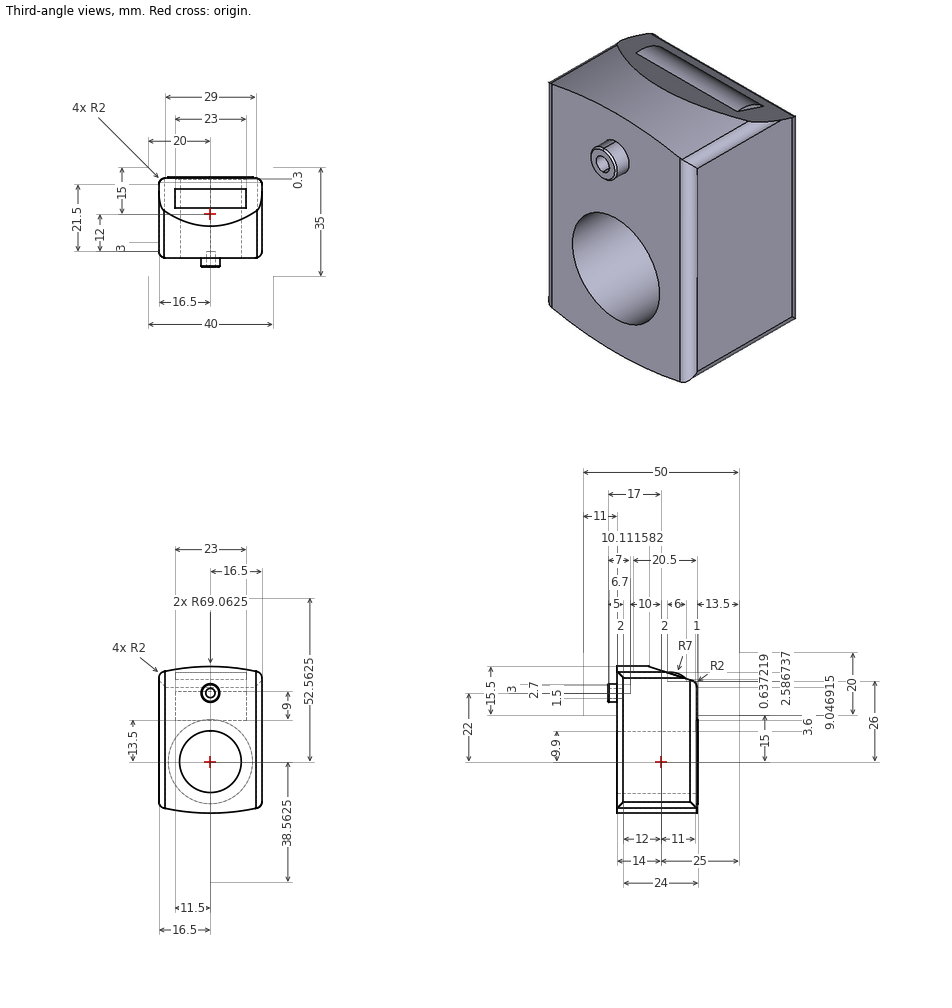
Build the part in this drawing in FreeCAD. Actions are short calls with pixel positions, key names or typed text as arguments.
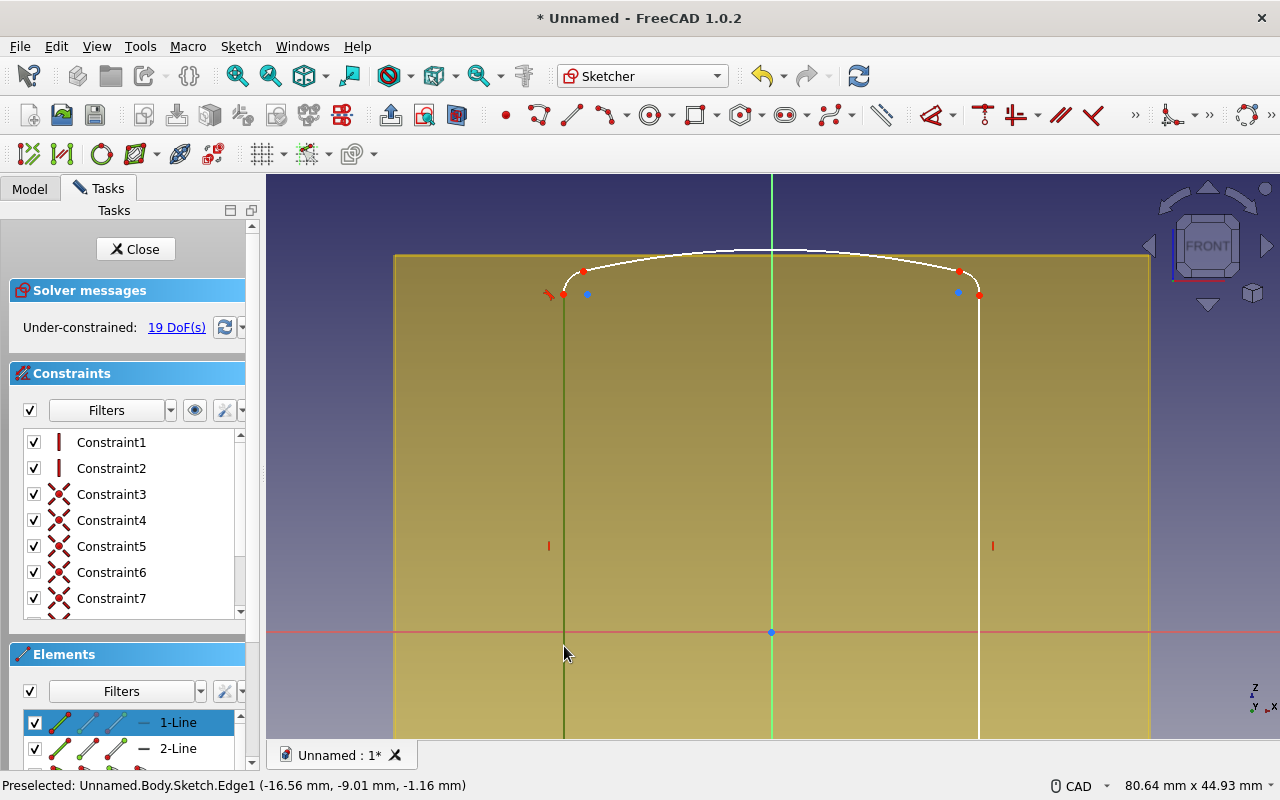
scroll(567, 278, down, 2)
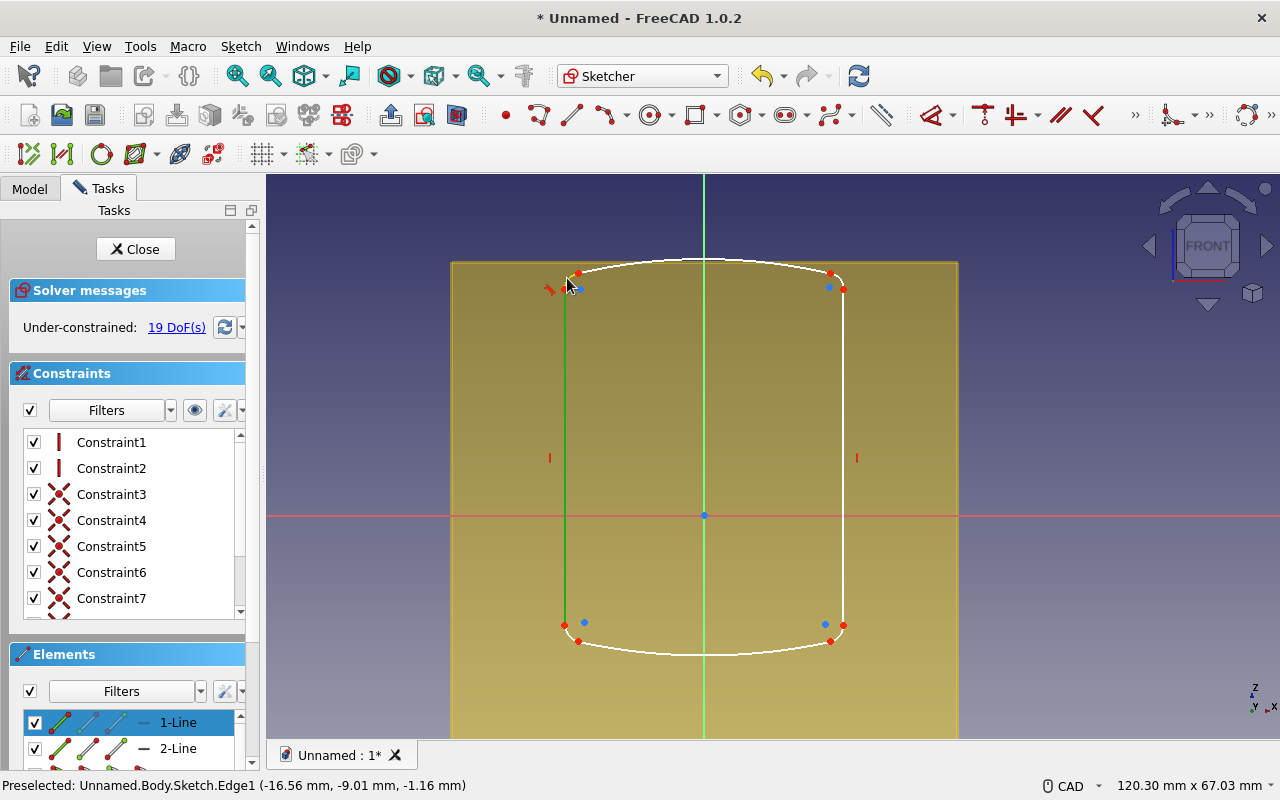
scroll(567, 632, up, 4)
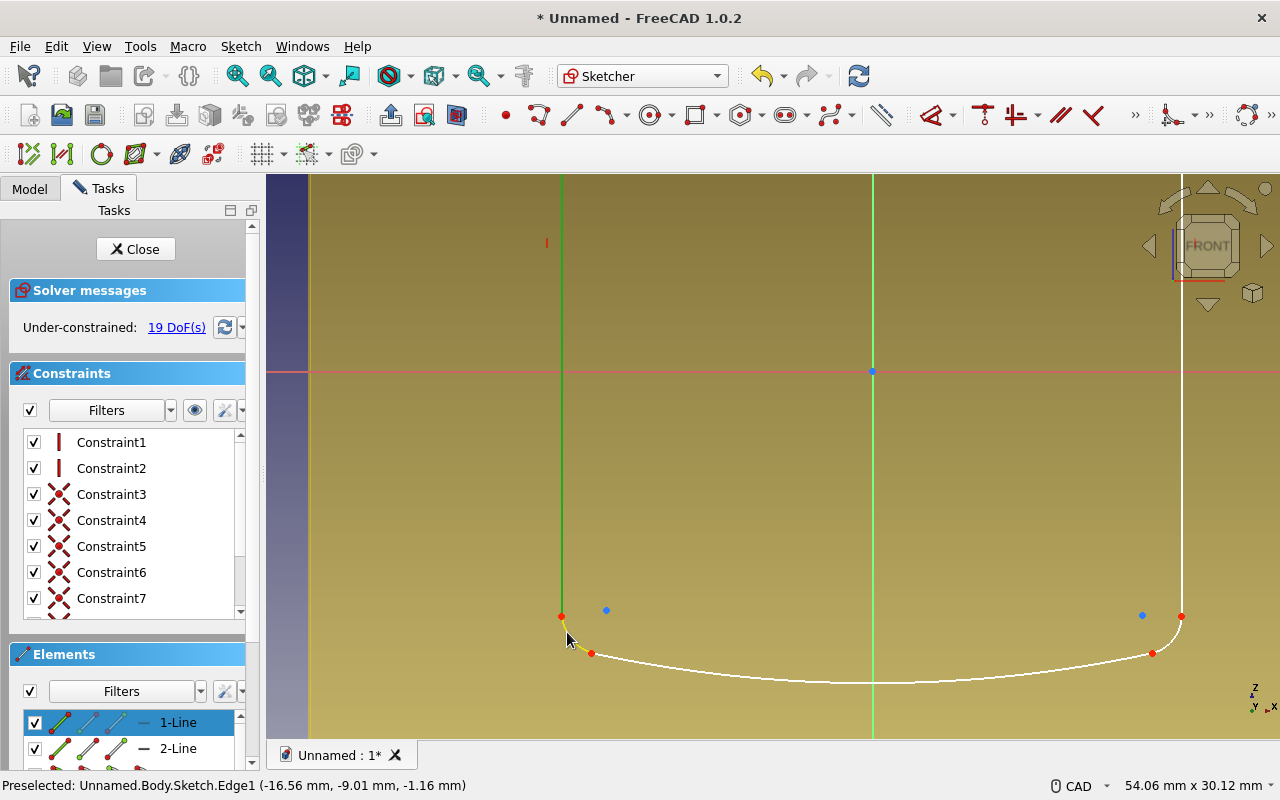
click(566, 631)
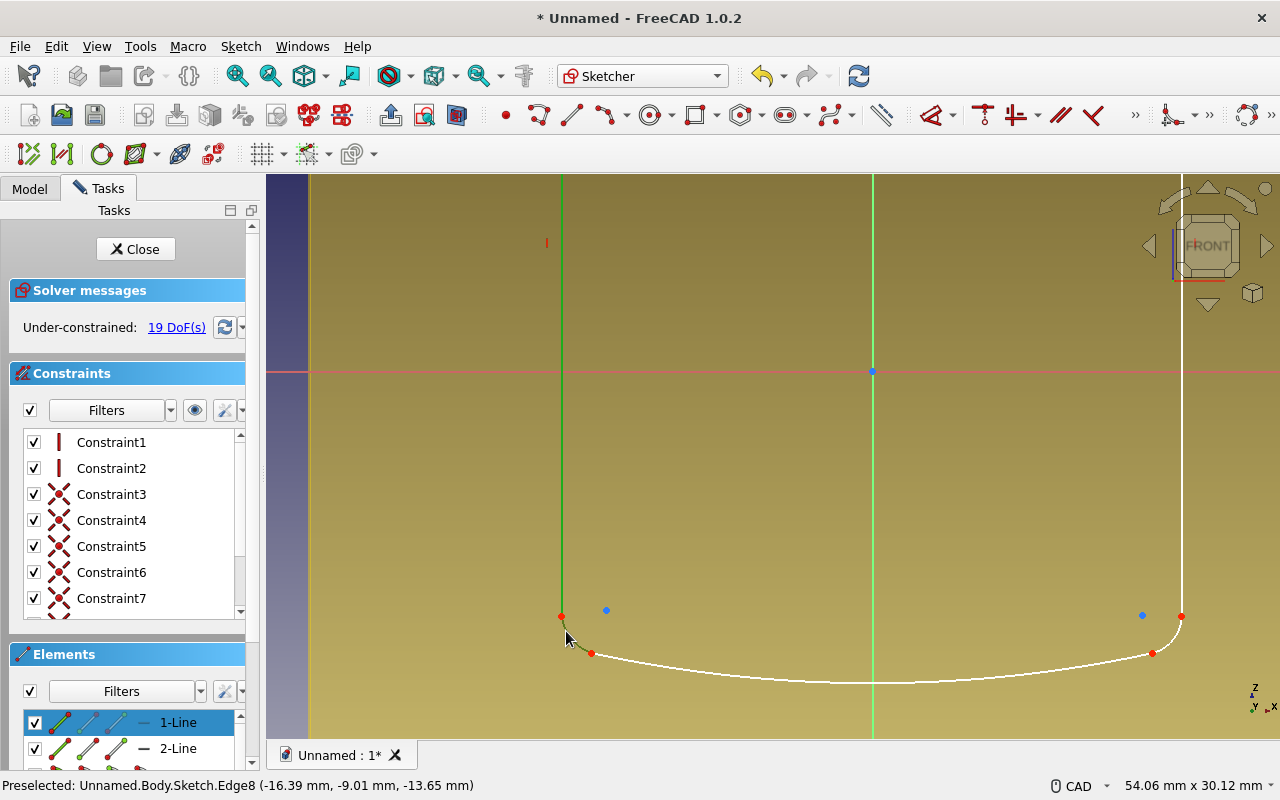
key(t)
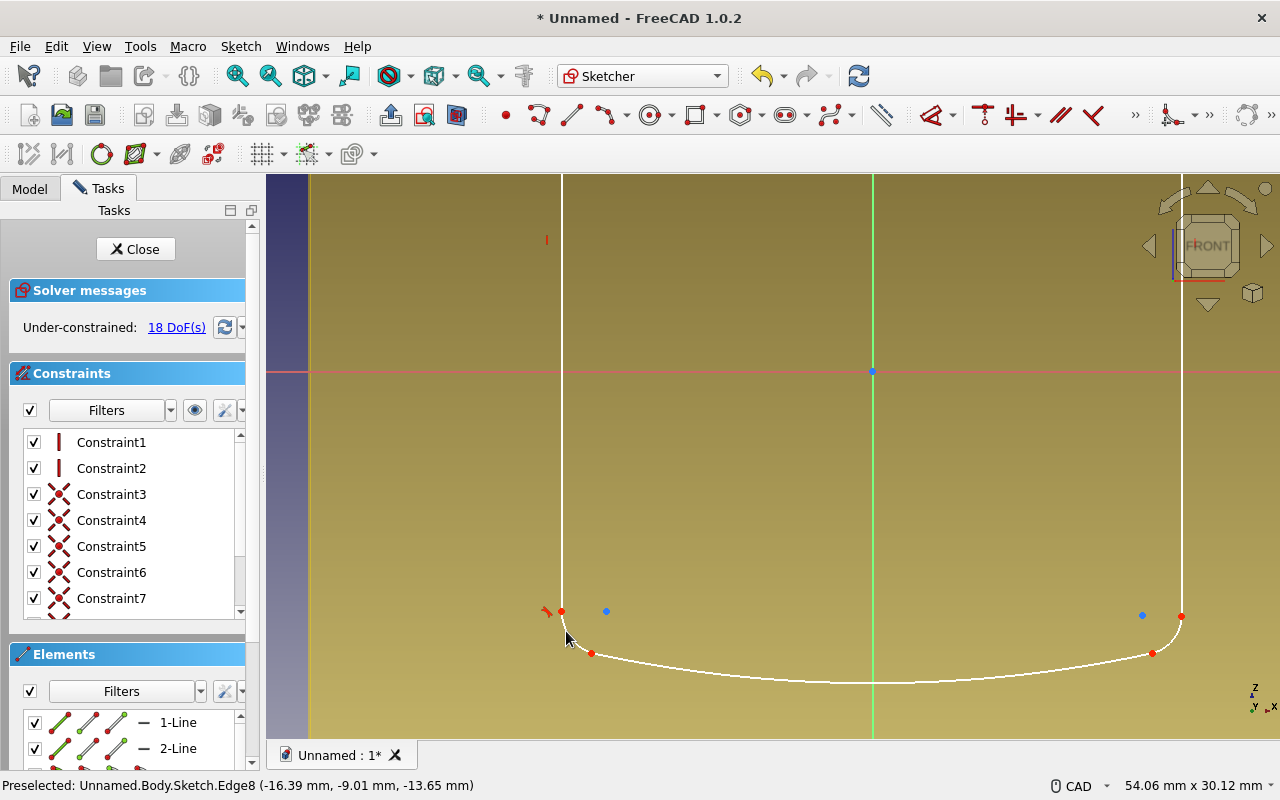
scroll(567, 633, down, 4)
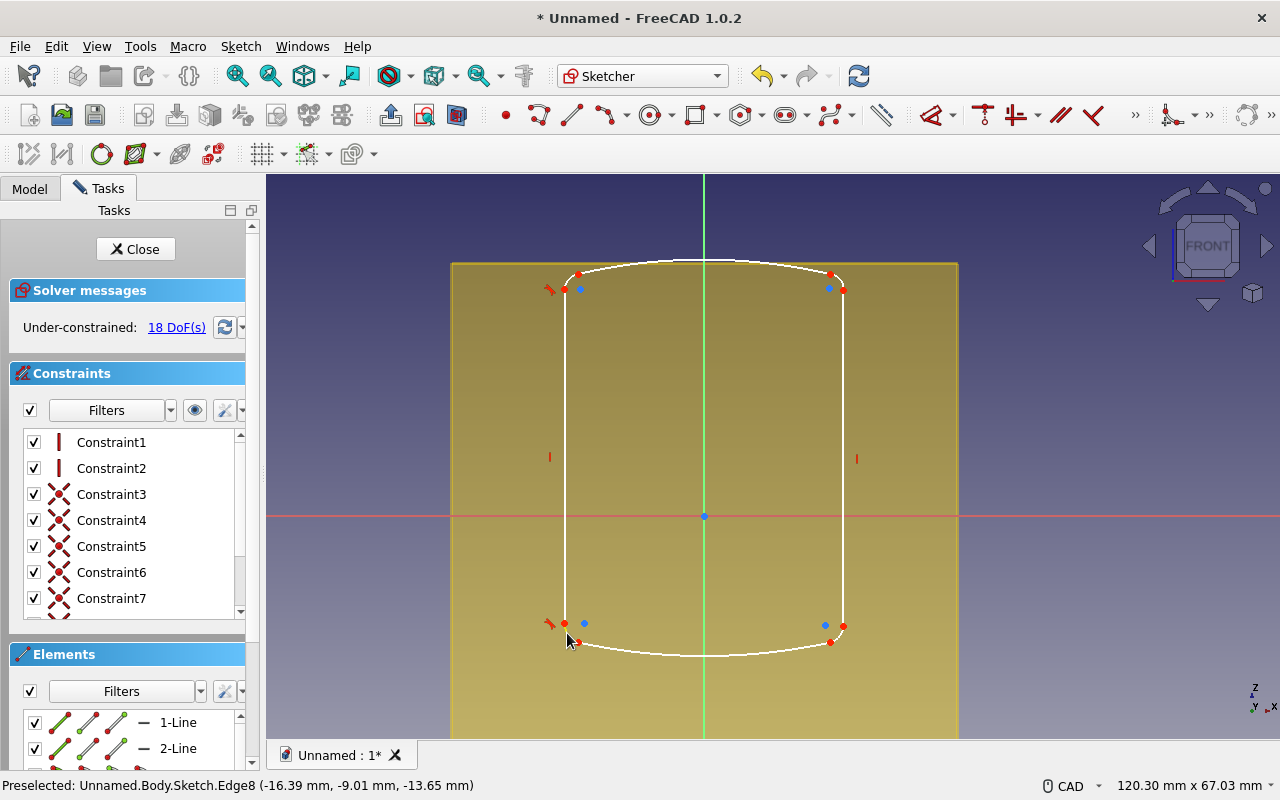
click(843, 391)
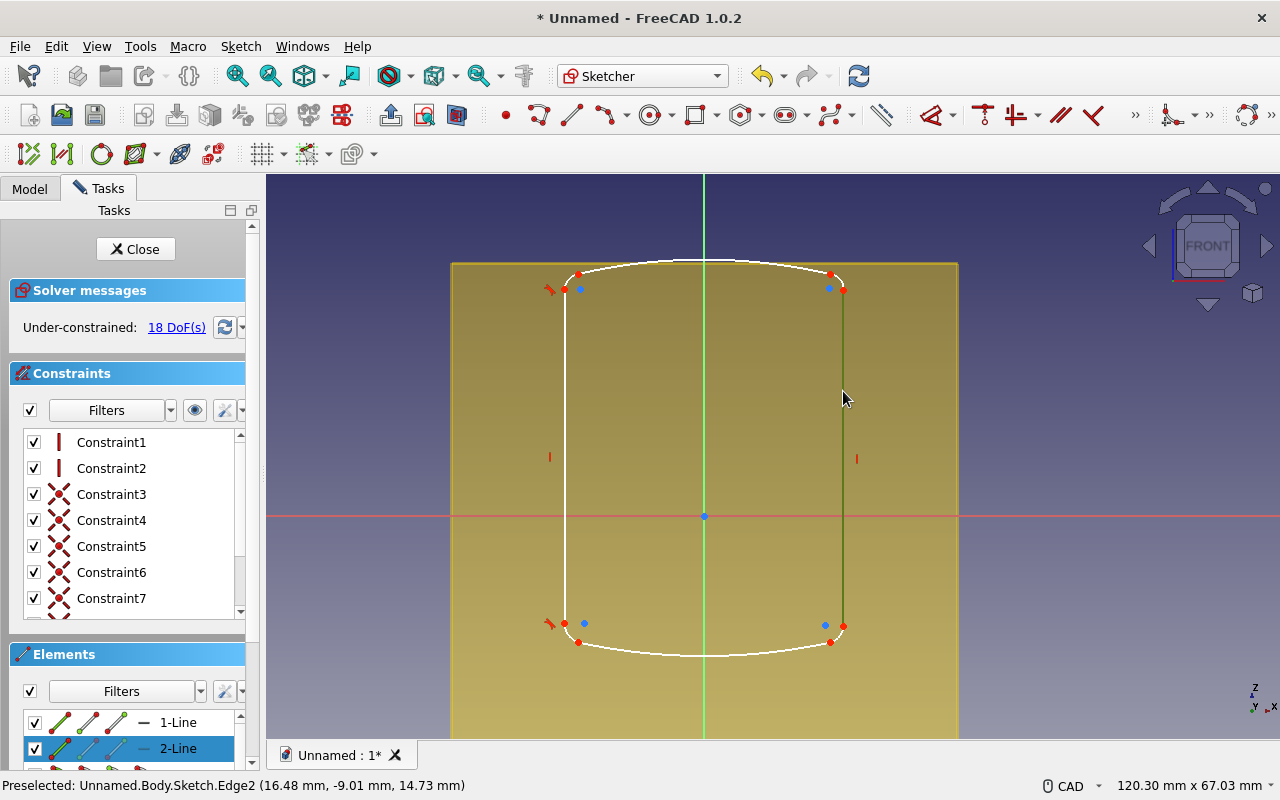
scroll(840, 279, up, 2)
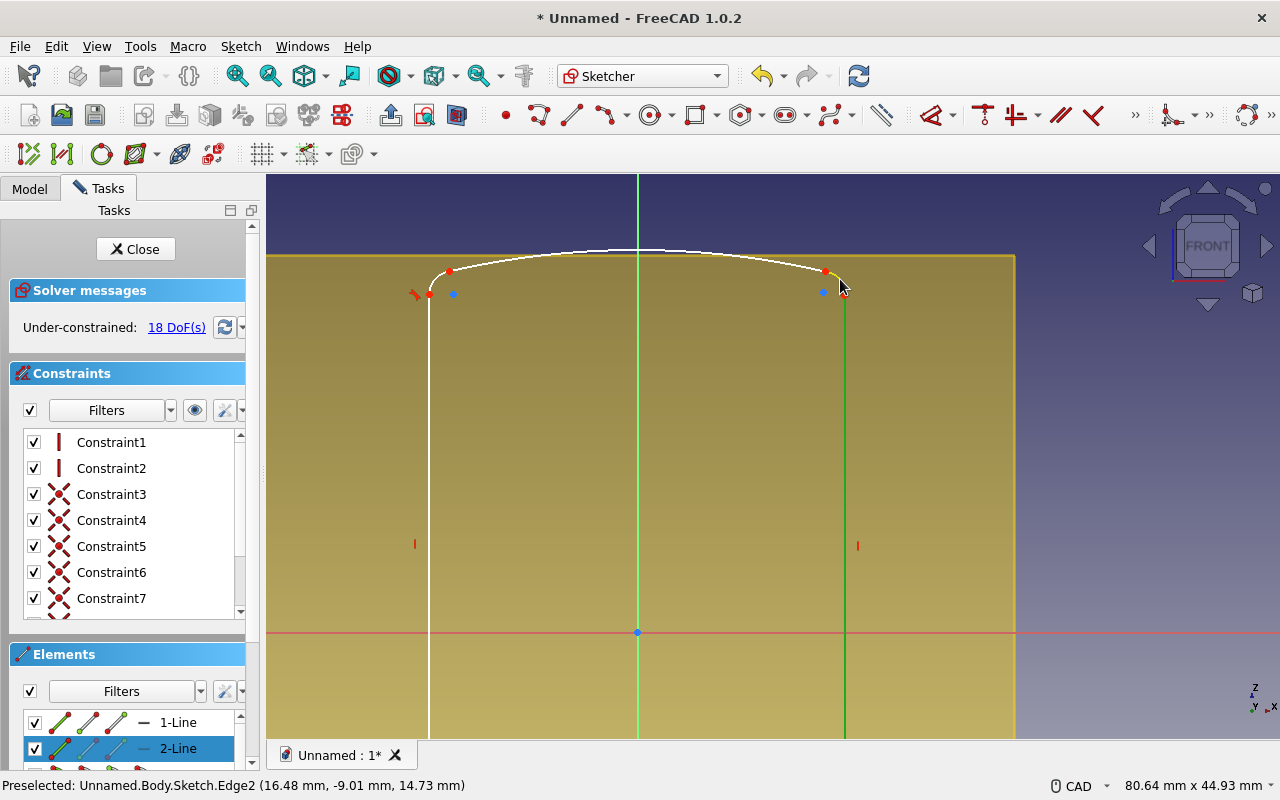
click(840, 279)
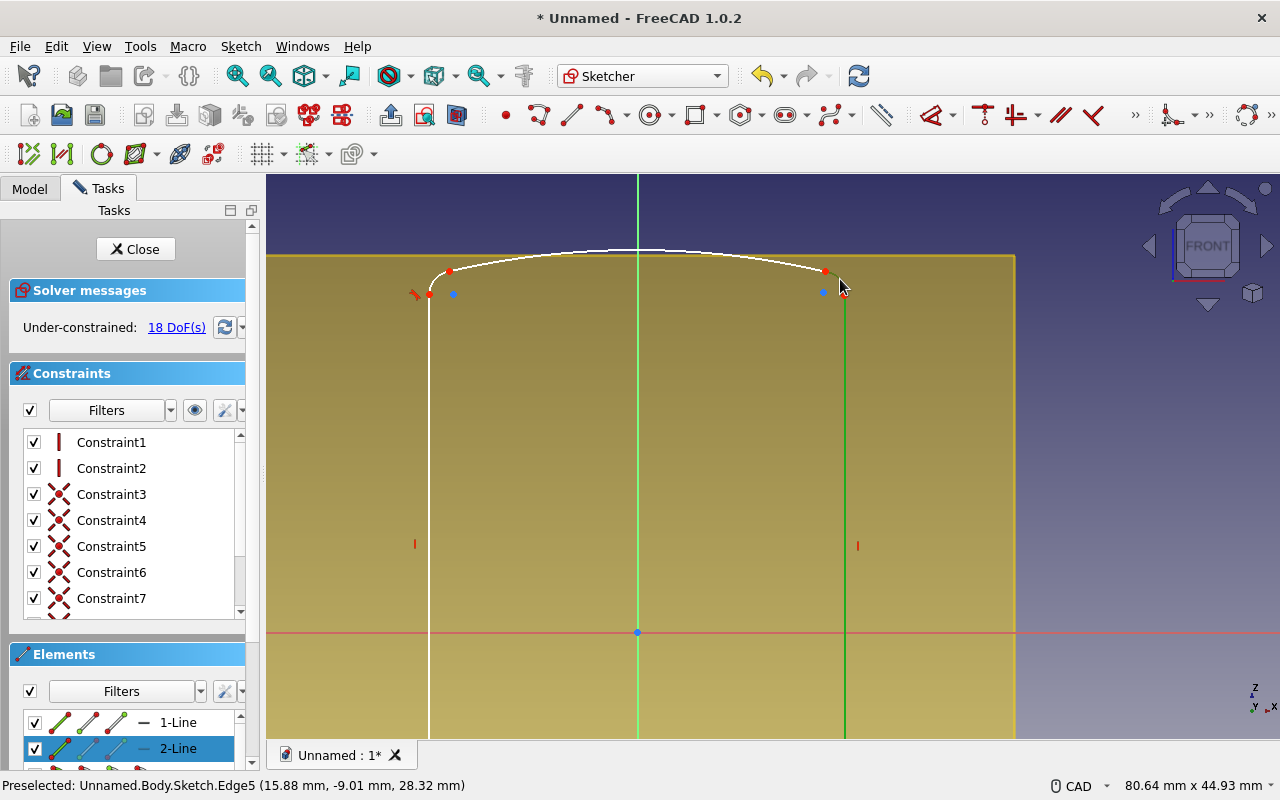
key(t)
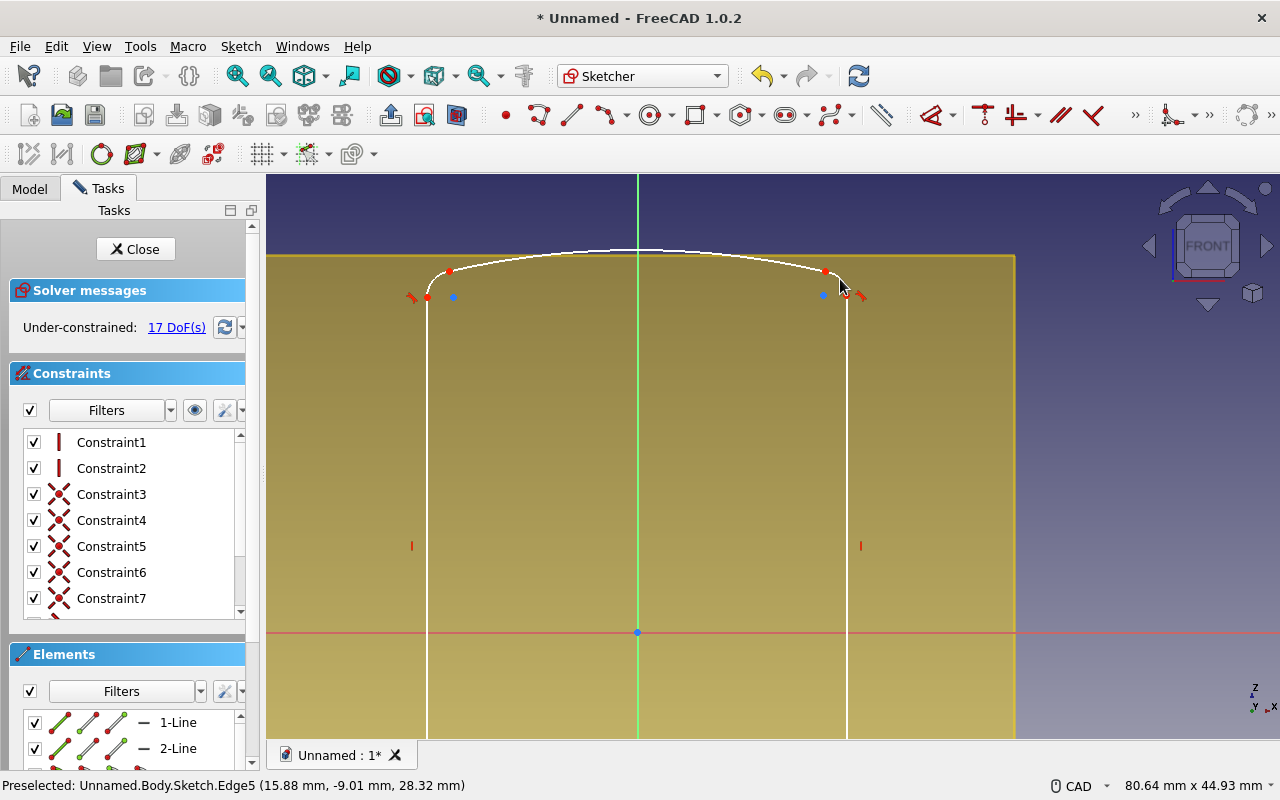
click(847, 446)